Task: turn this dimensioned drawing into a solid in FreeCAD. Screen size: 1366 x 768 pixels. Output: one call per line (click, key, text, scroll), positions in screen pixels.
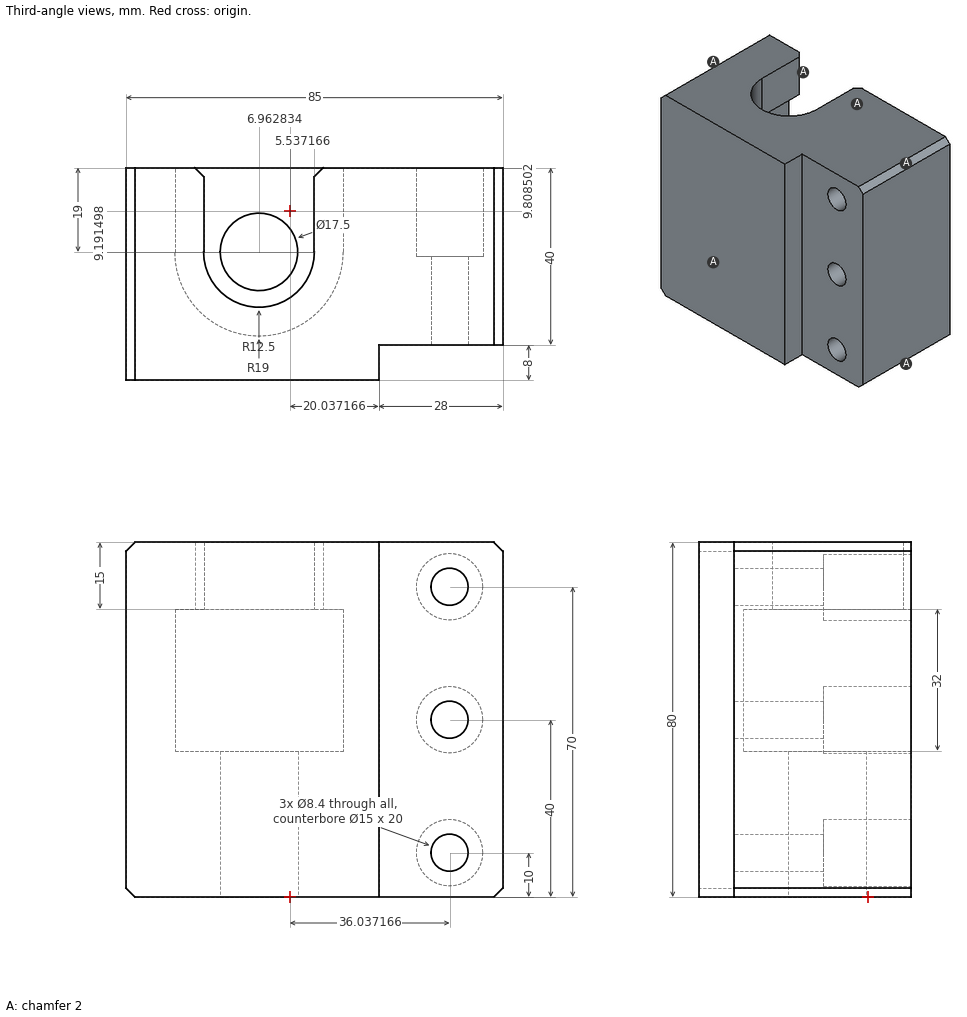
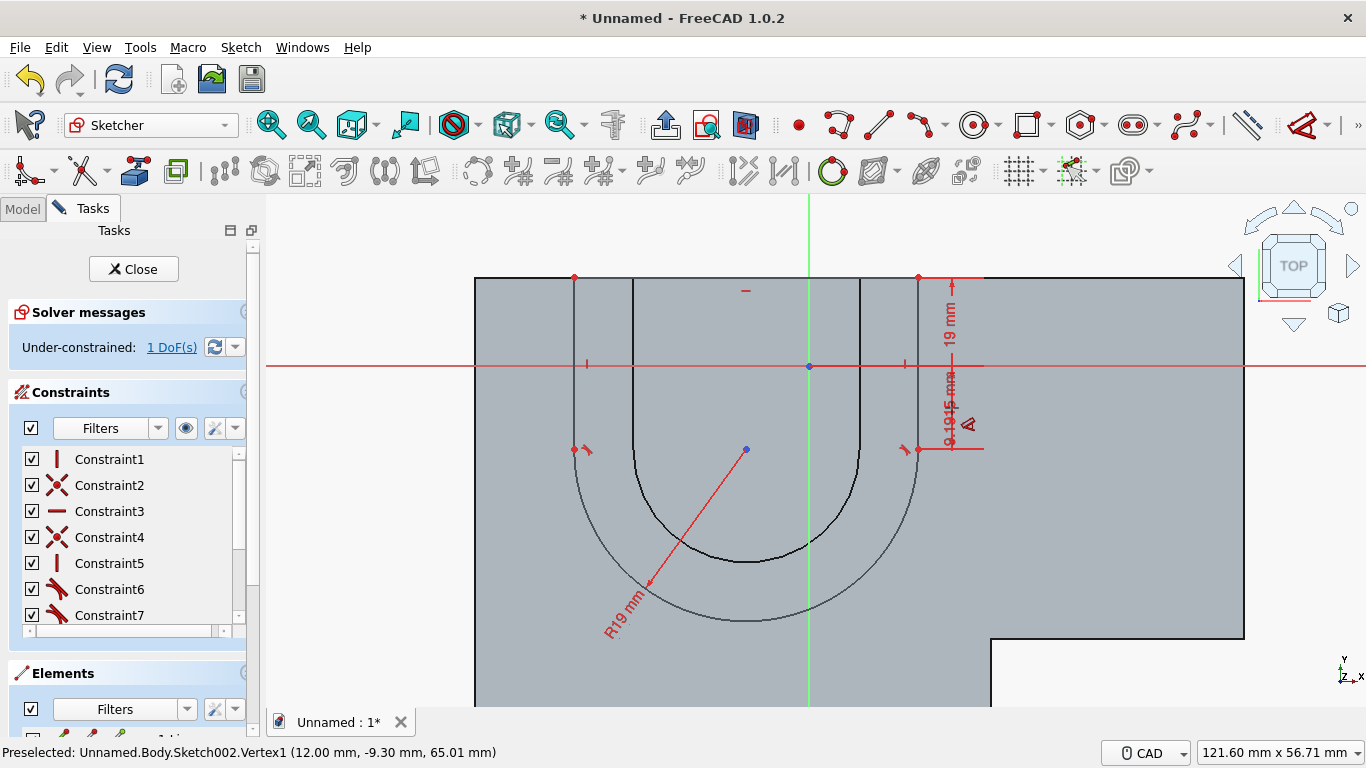
click(746, 449)
click(778, 332)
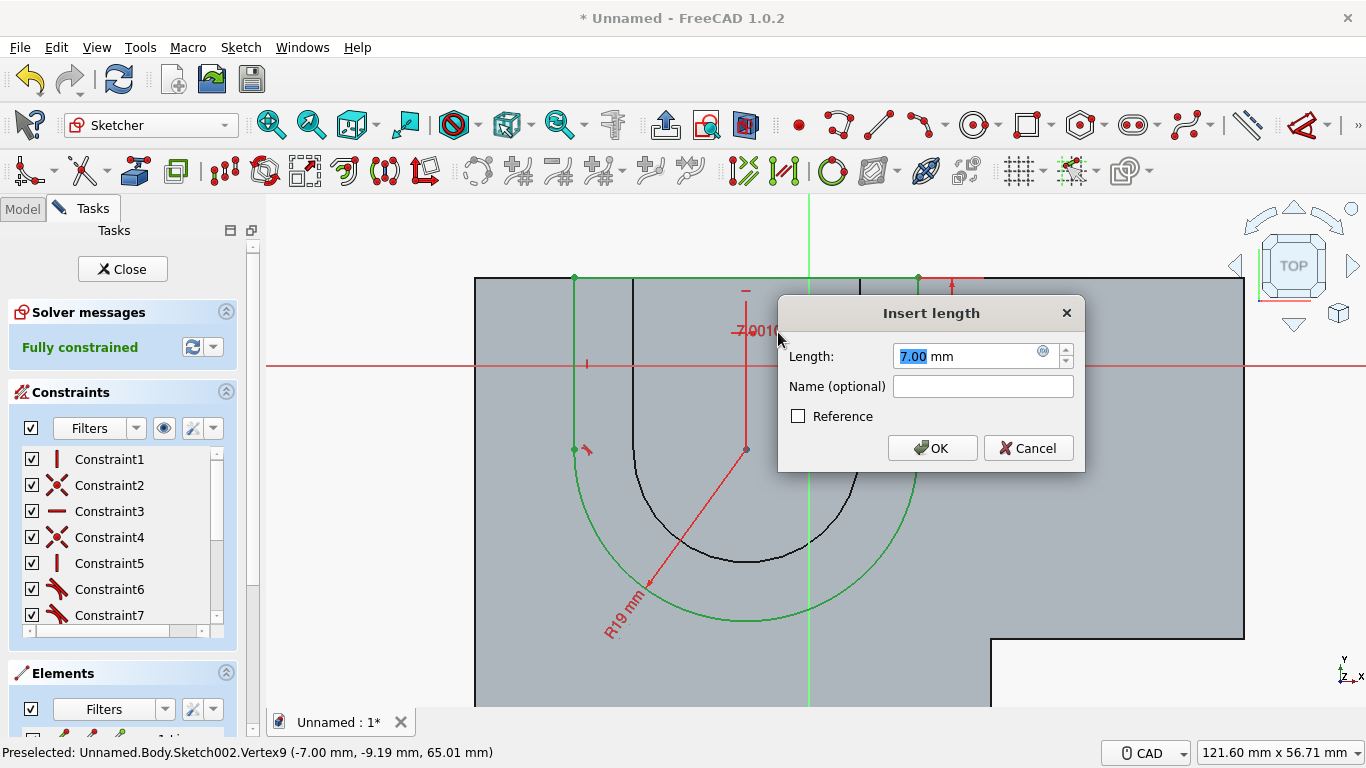
text(6.962834)
key(Return)
key(Escape)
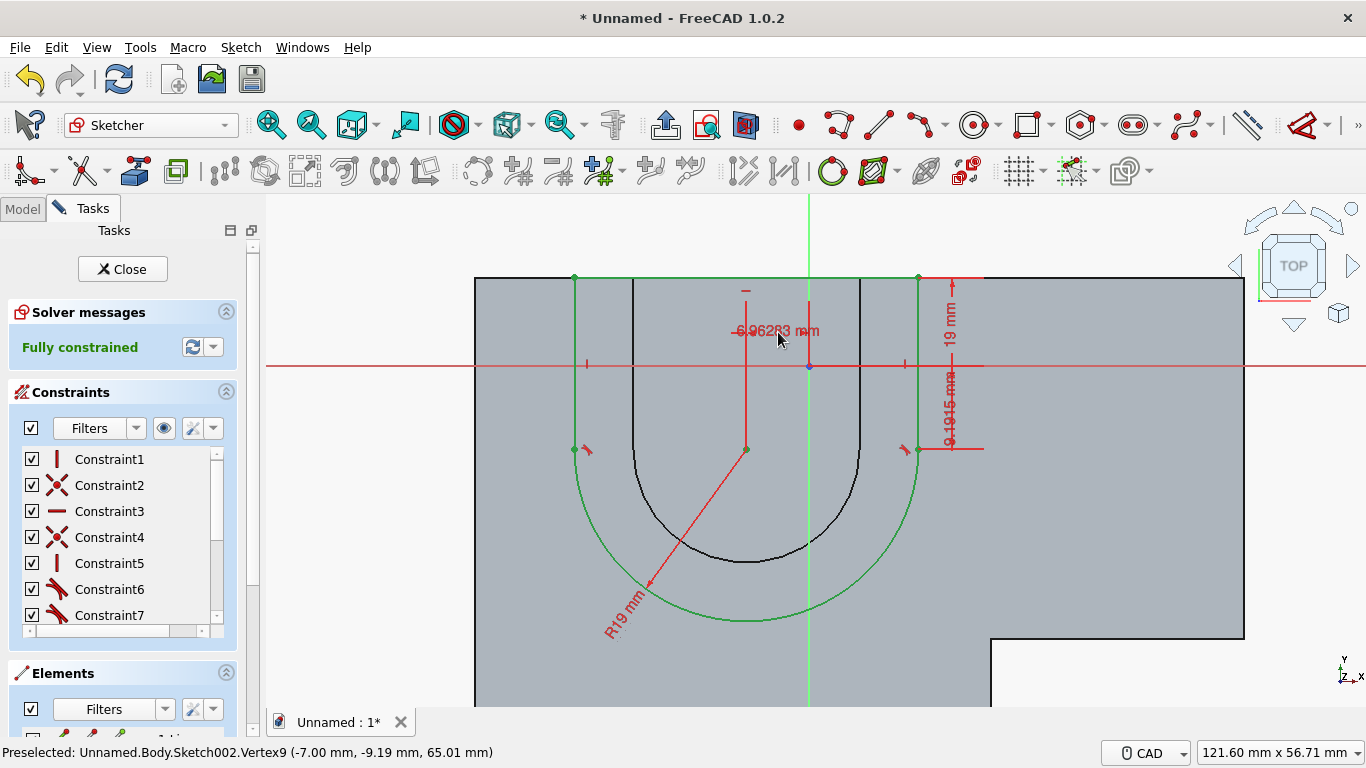
click(123, 269)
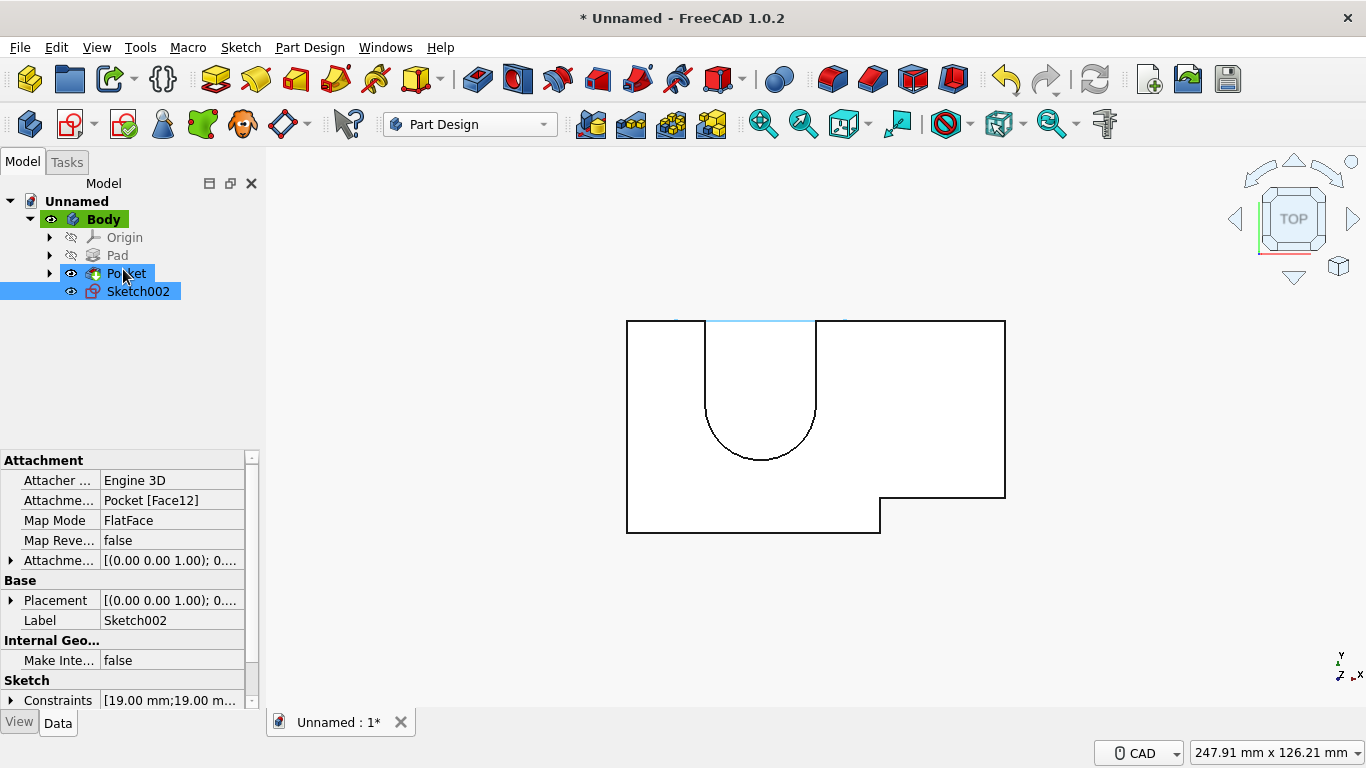
click(478, 80)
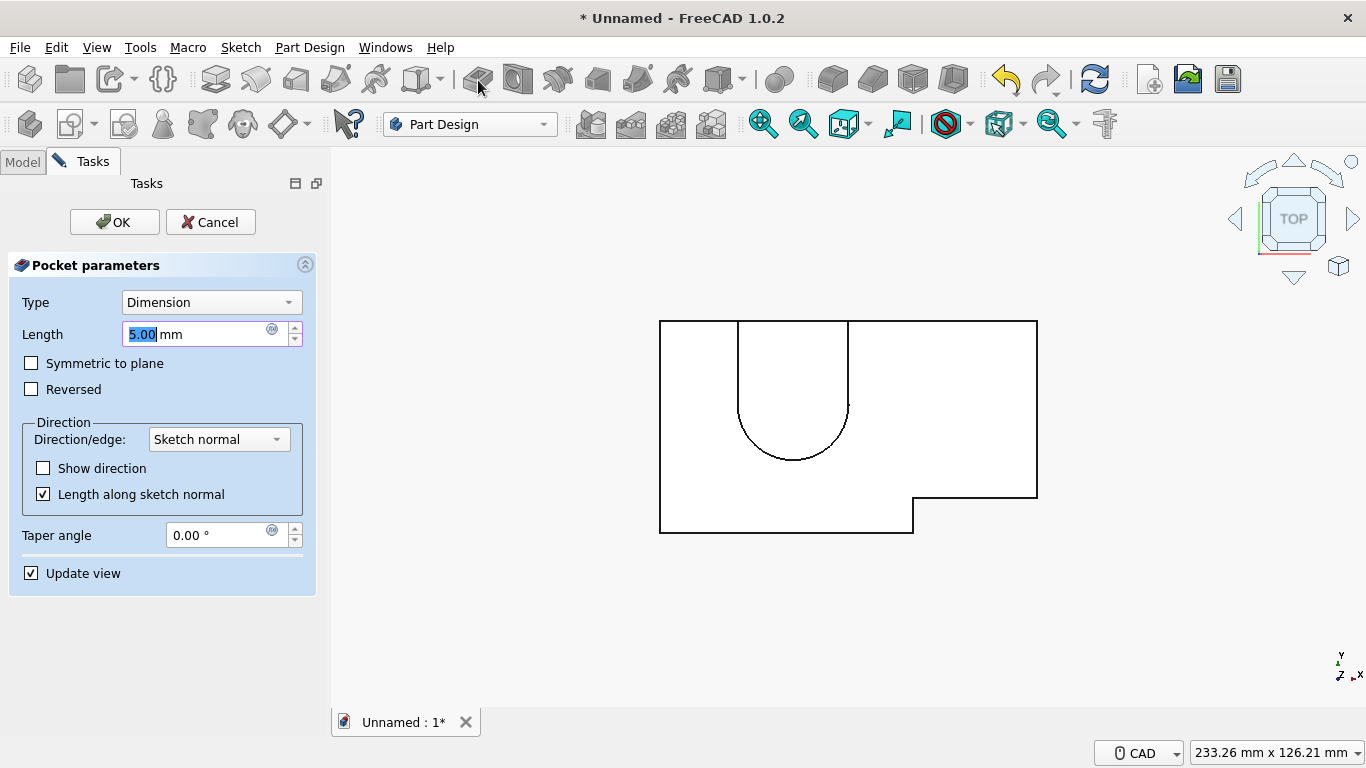
text(32)
key(Tab)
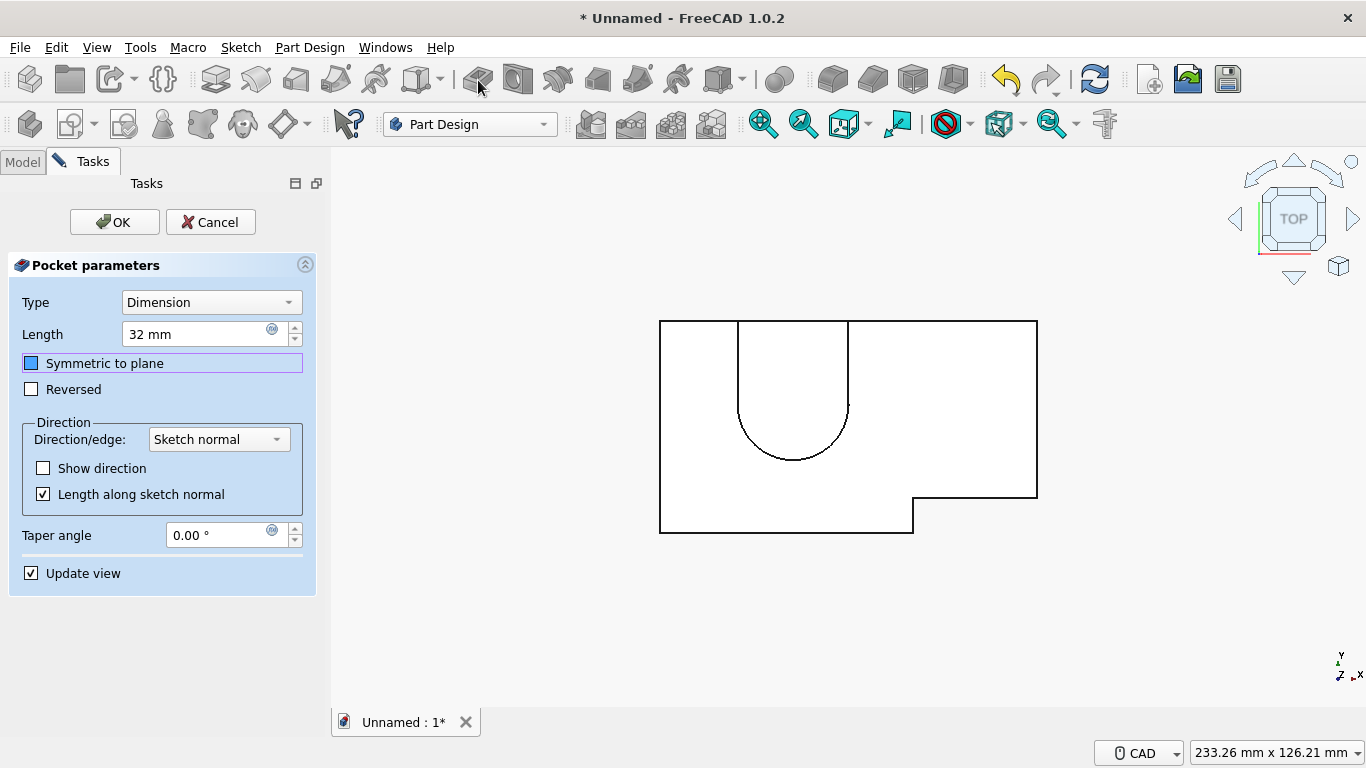
click(115, 222)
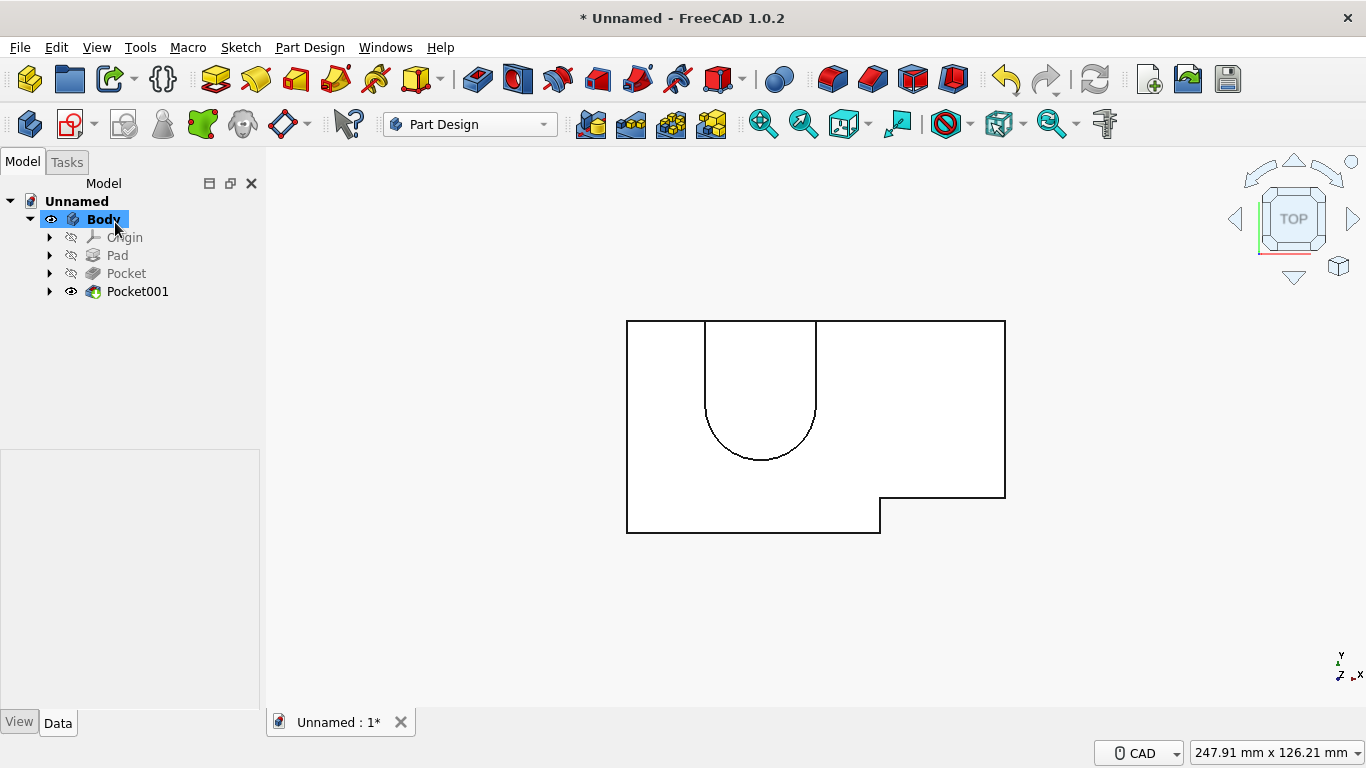
click(764, 124)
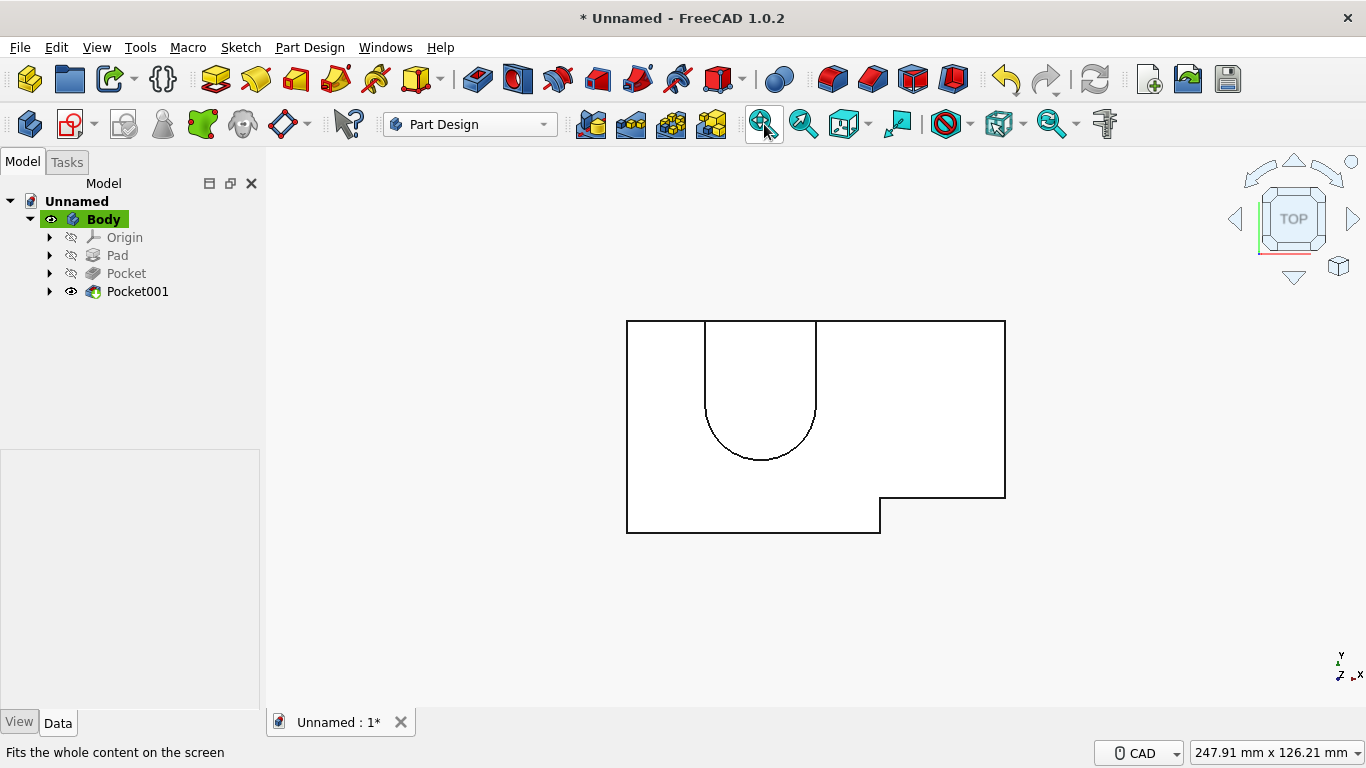
click(761, 404)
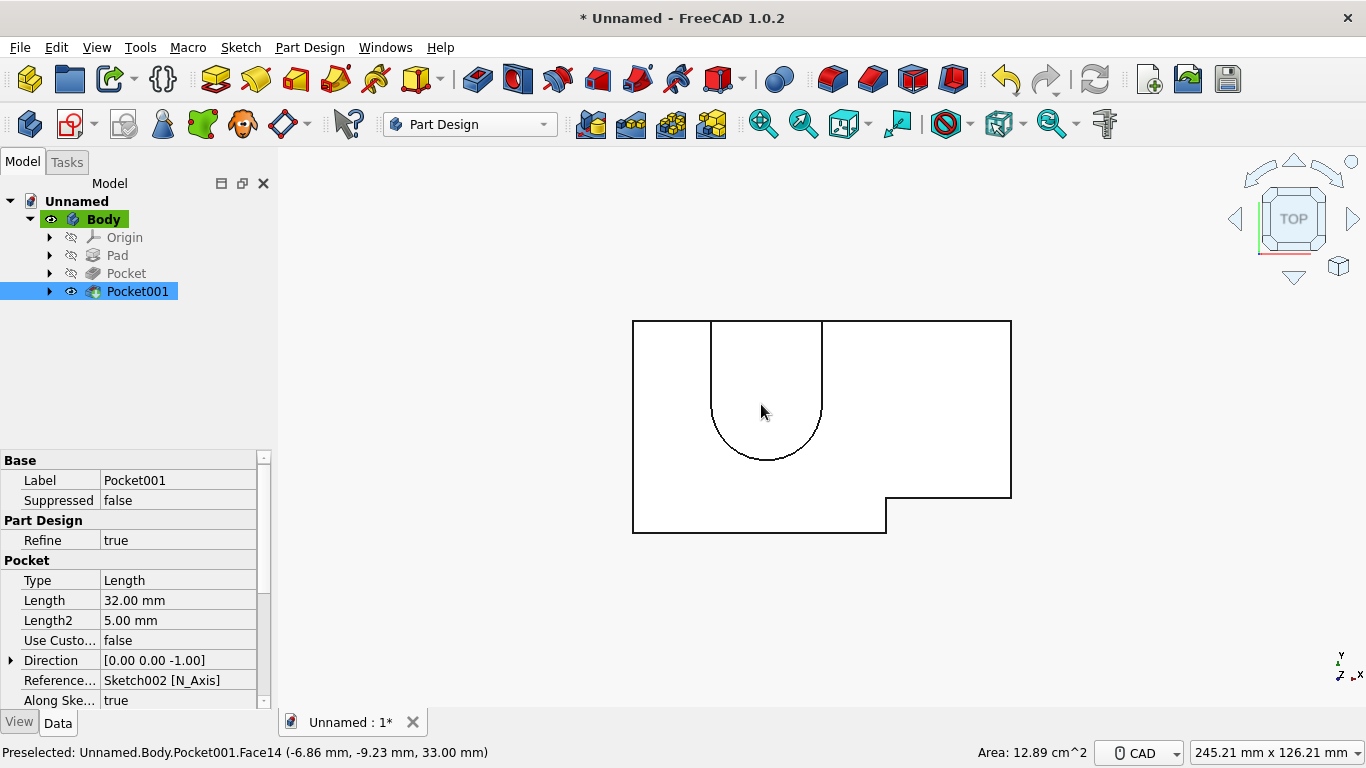
click(70, 124)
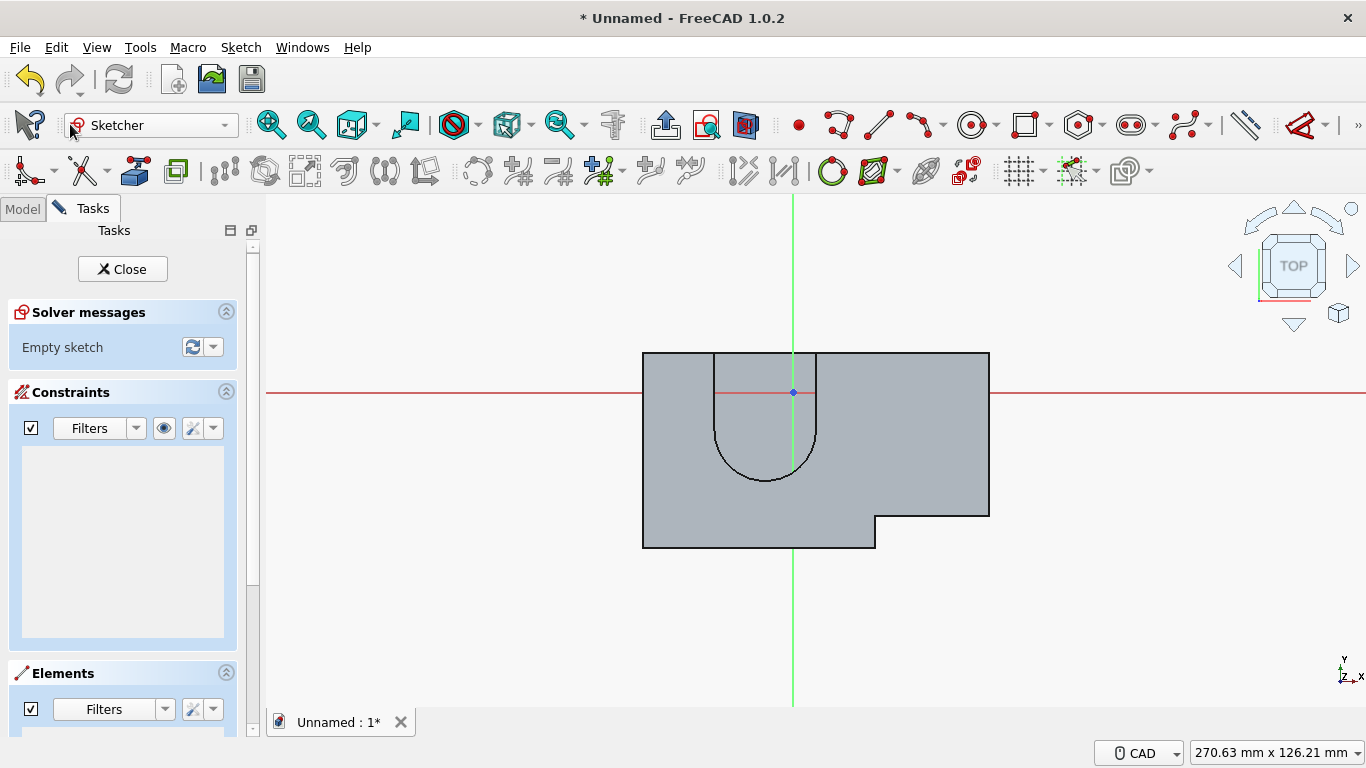
click(746, 126)